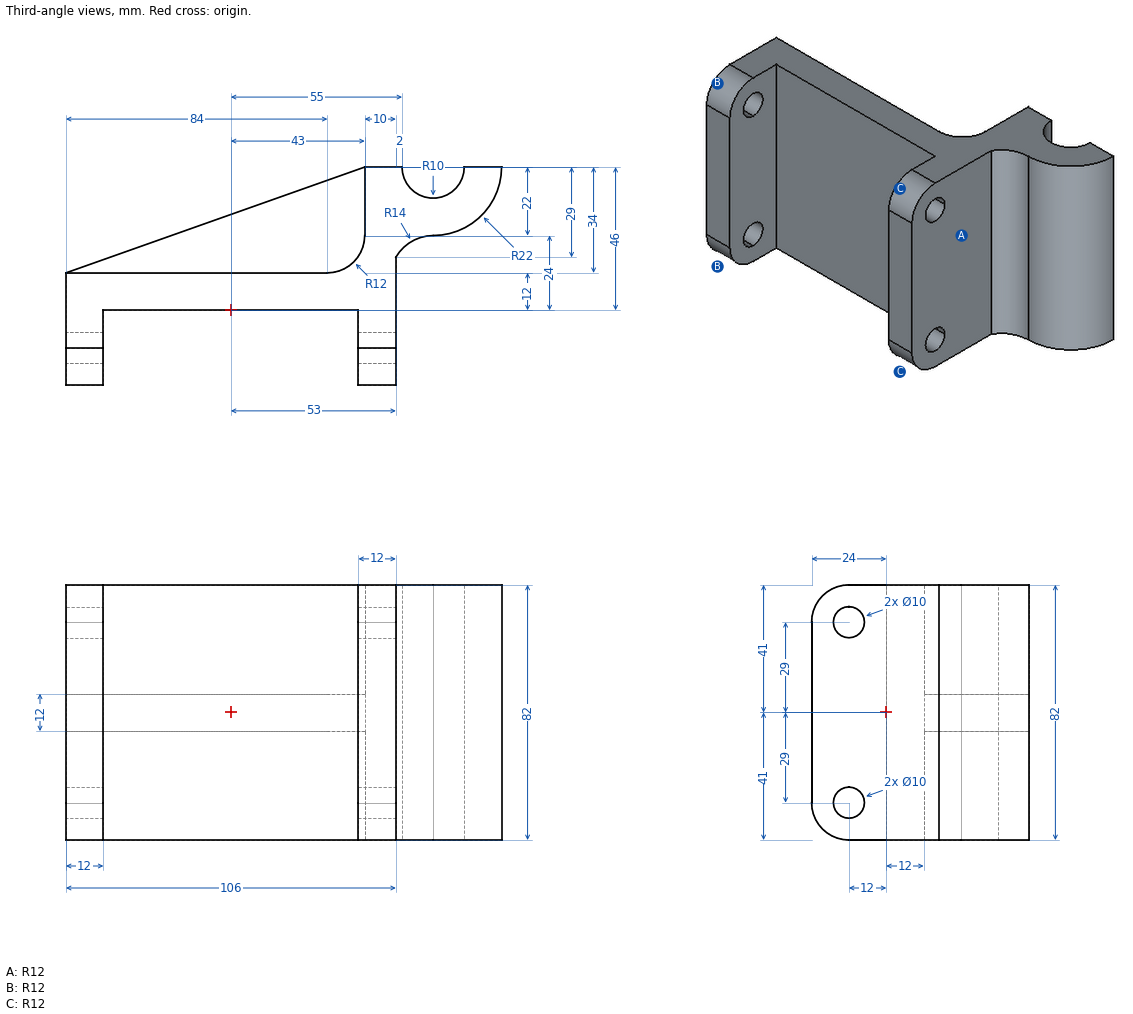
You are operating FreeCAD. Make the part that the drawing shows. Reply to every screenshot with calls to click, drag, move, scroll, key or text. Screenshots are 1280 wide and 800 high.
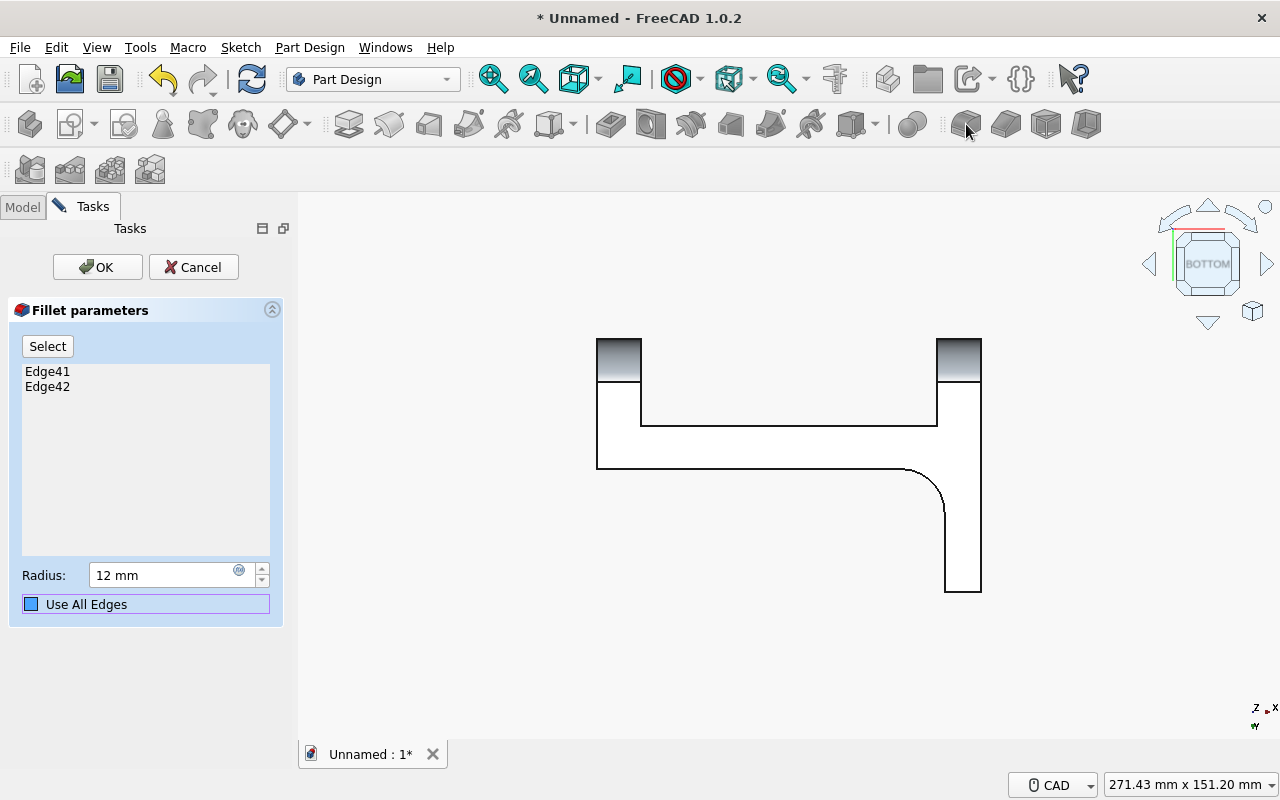
click(98, 267)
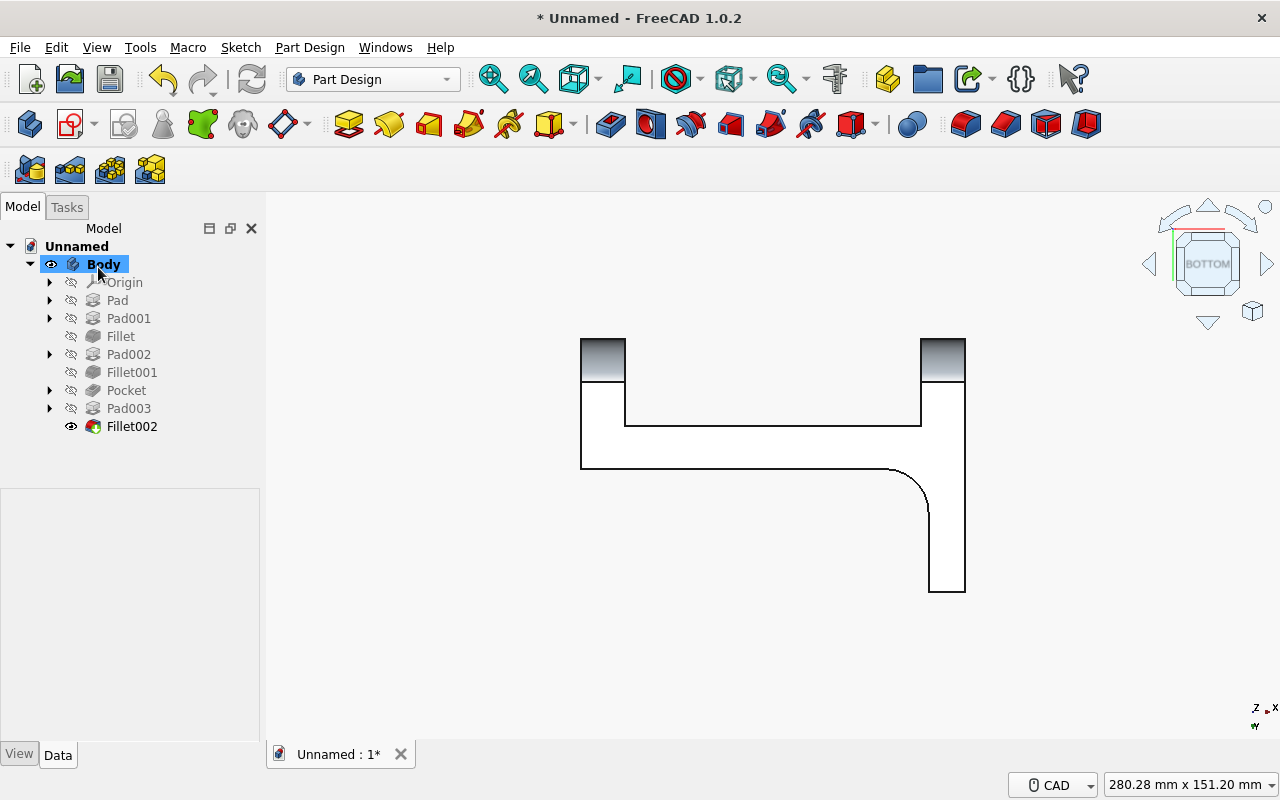
click(50, 282)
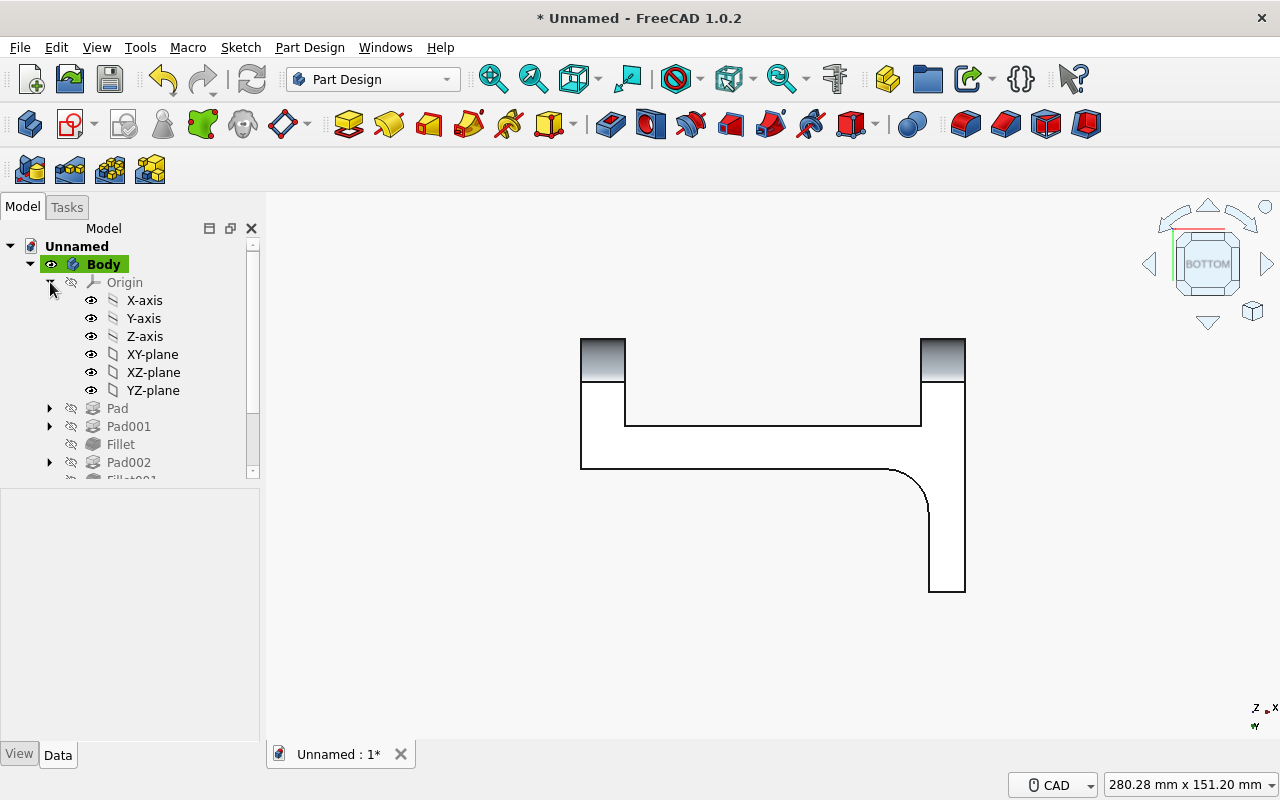
click(136, 390)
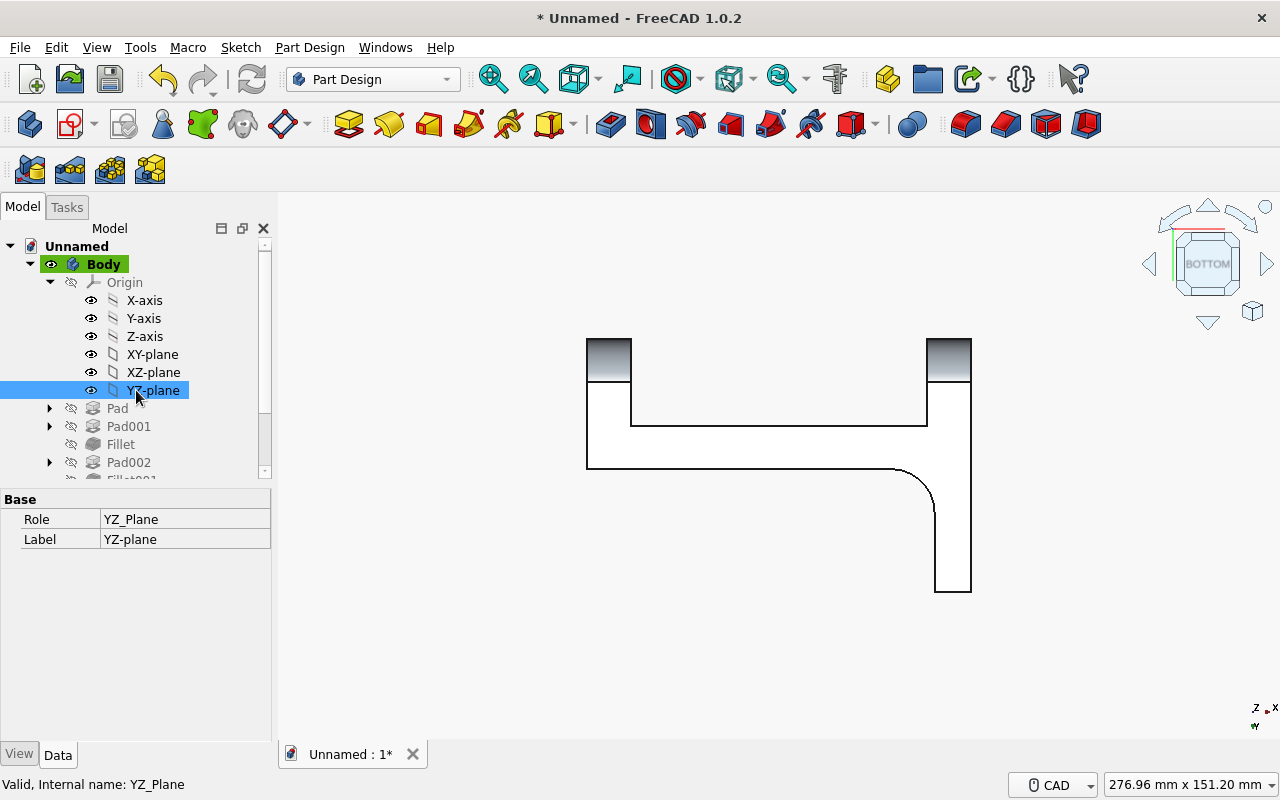
click(284, 124)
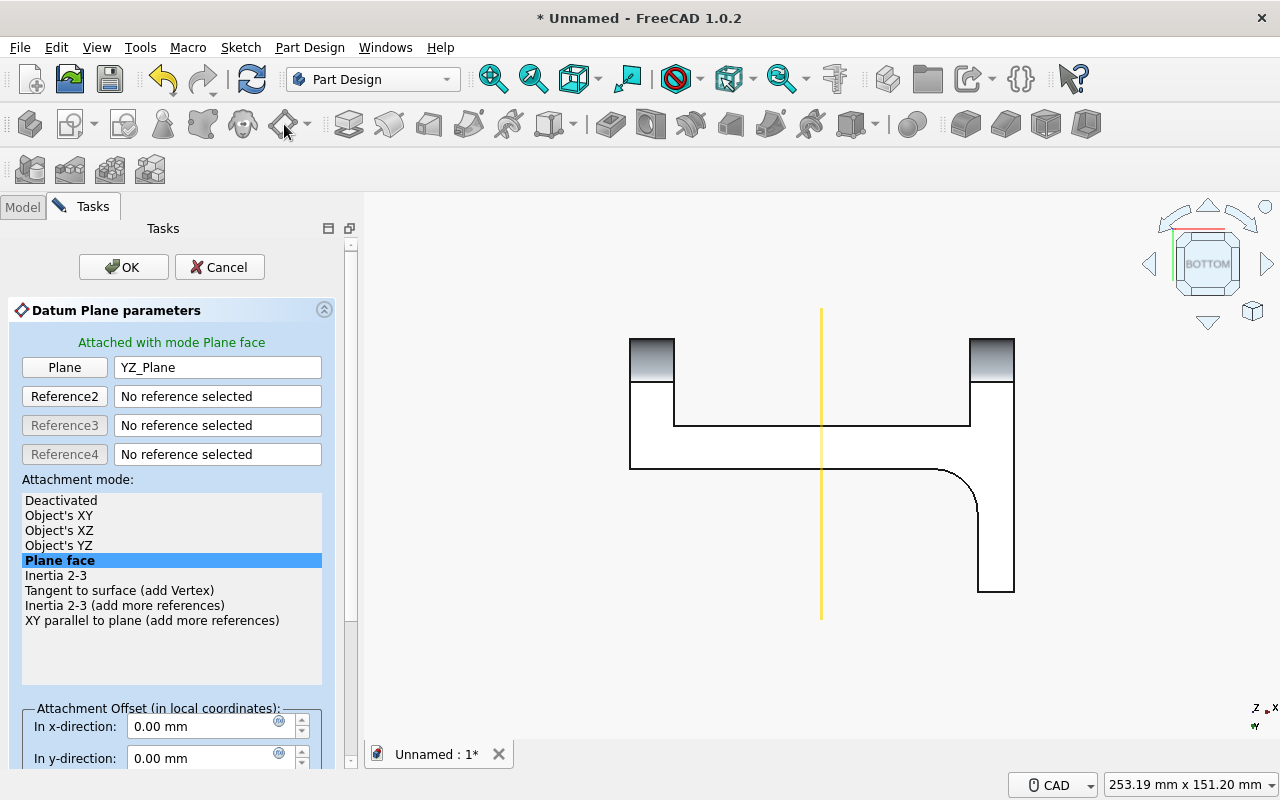
scroll(351, 503, down, 2)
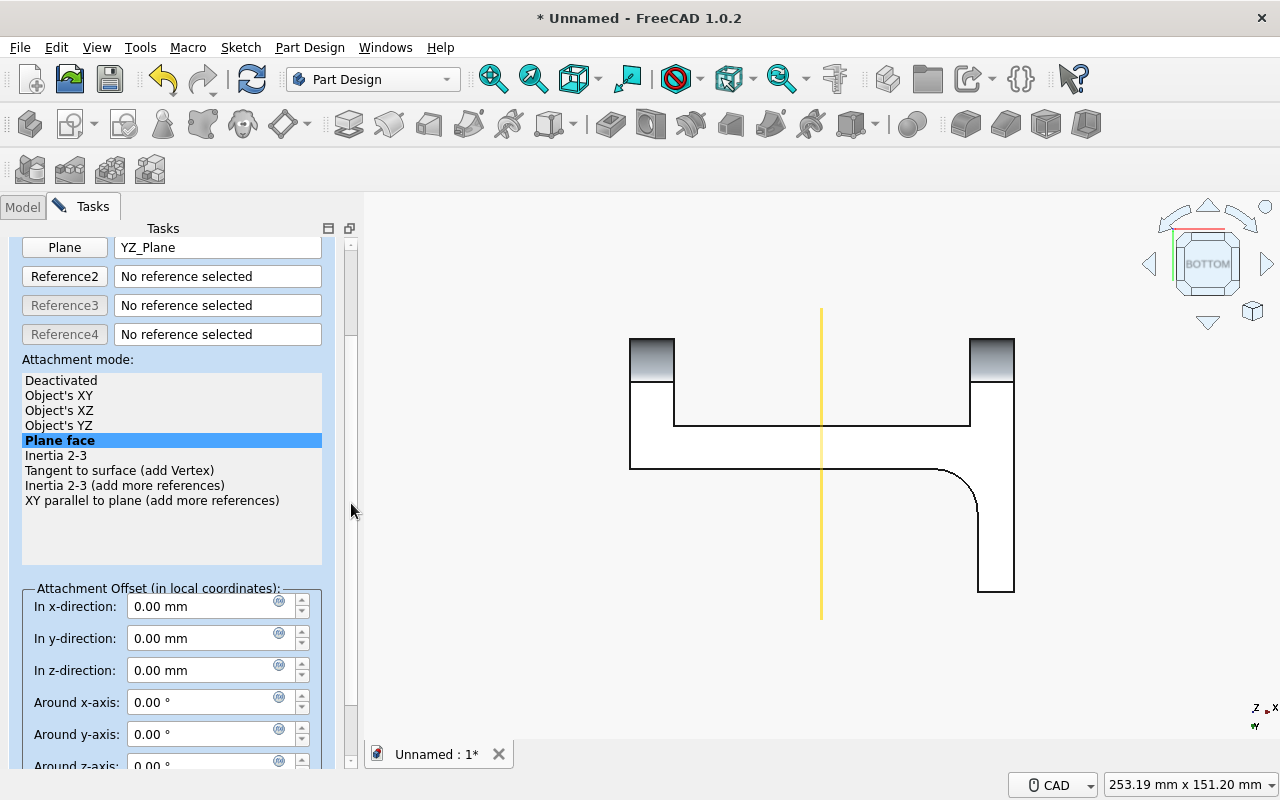
triple_click(210, 670)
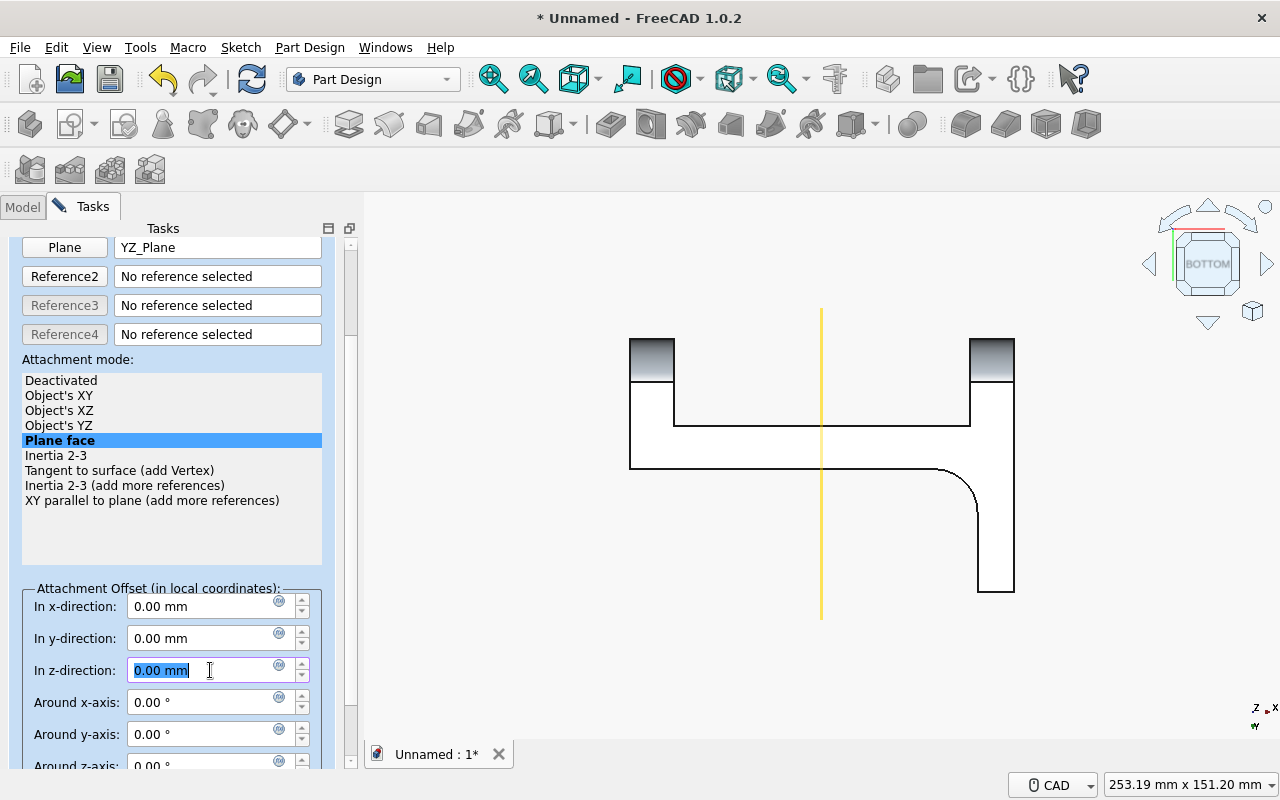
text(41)
key(Tab)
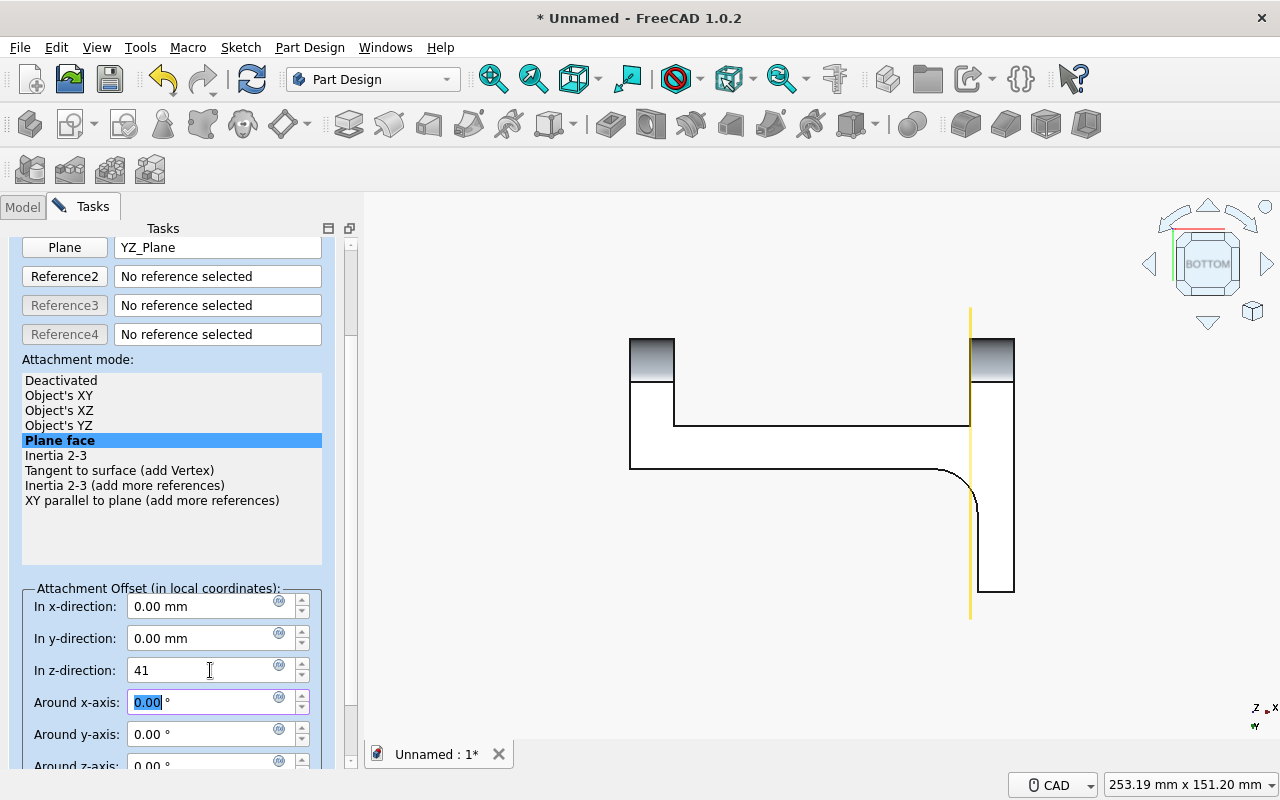
scroll(351, 503, up, 3)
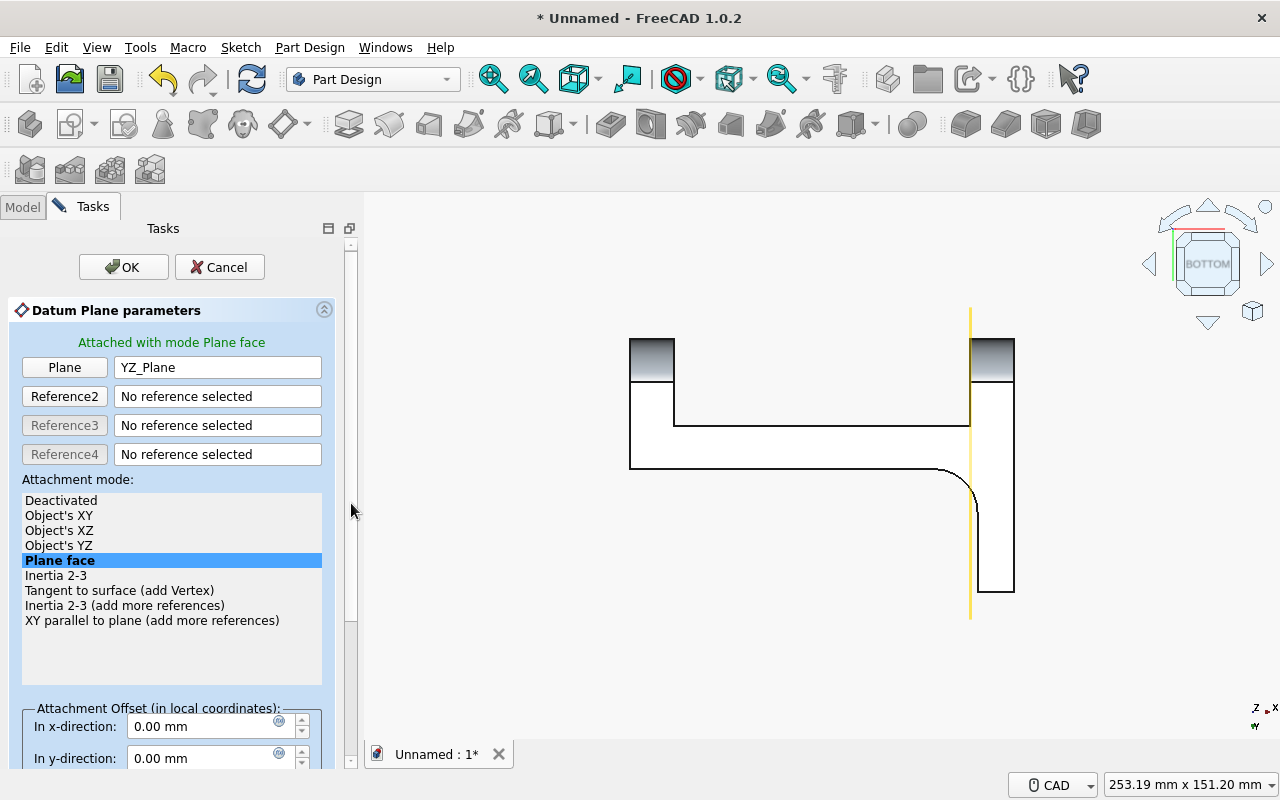
click(124, 267)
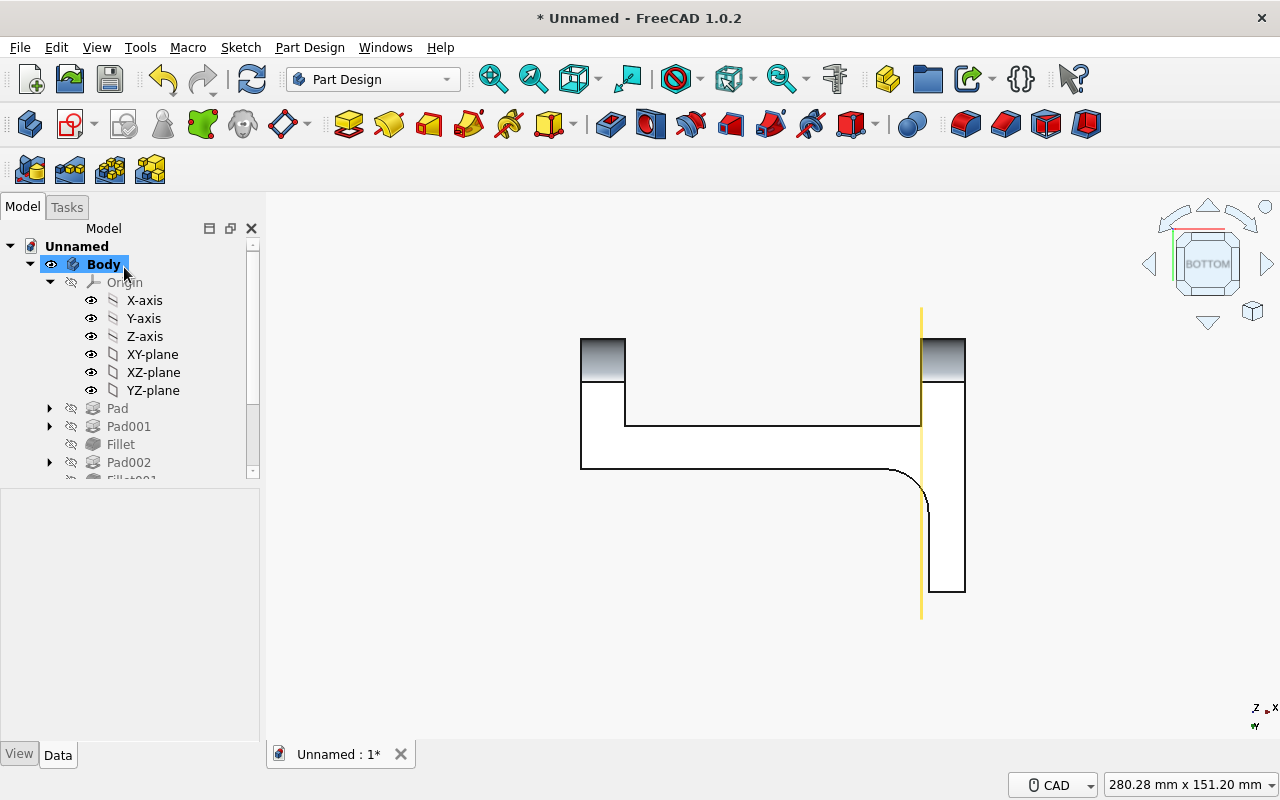
scroll(100, 350, down, 3)